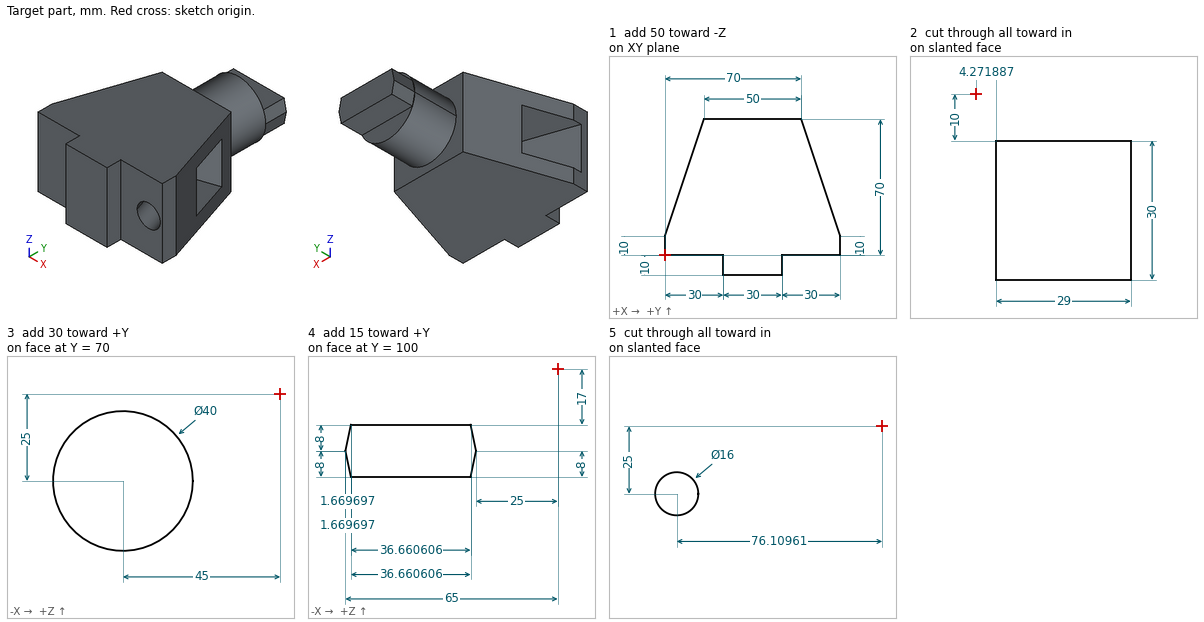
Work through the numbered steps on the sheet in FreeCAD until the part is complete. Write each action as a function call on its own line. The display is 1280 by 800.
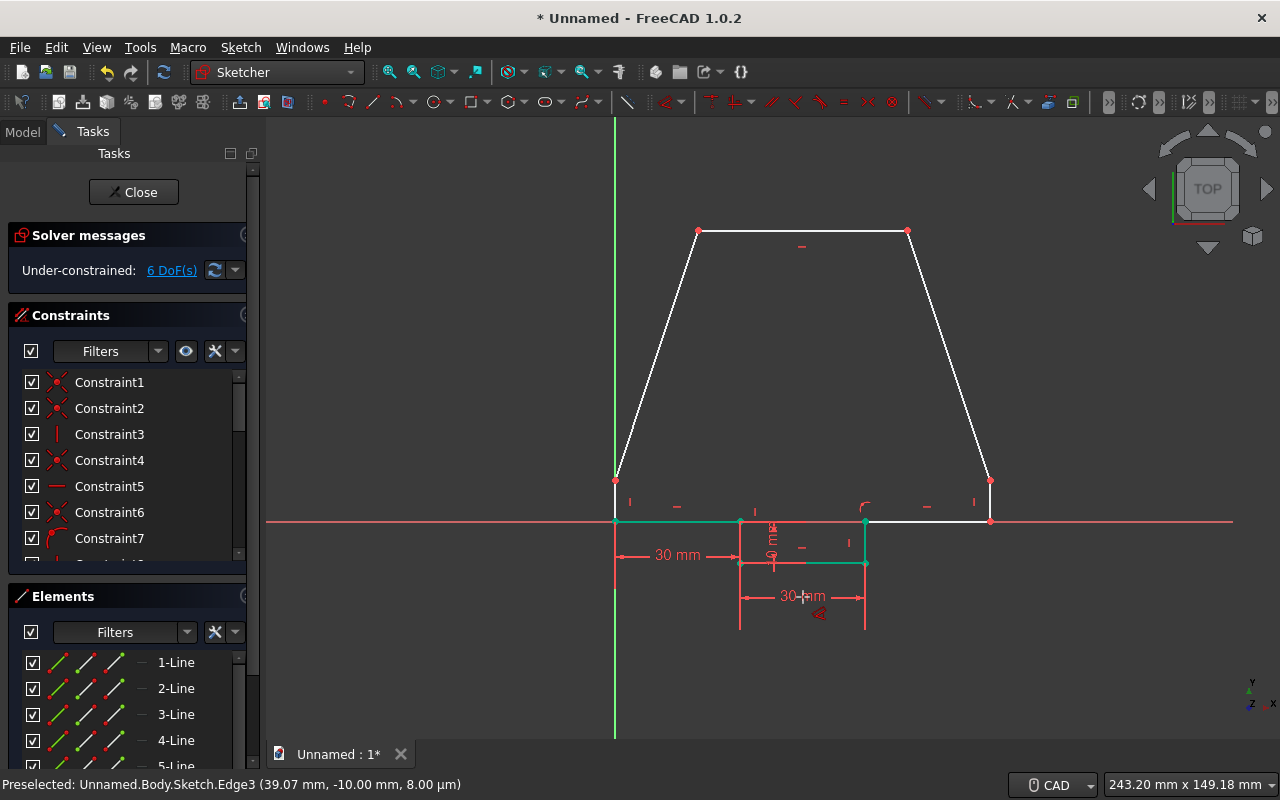
click(903, 522)
click(928, 556)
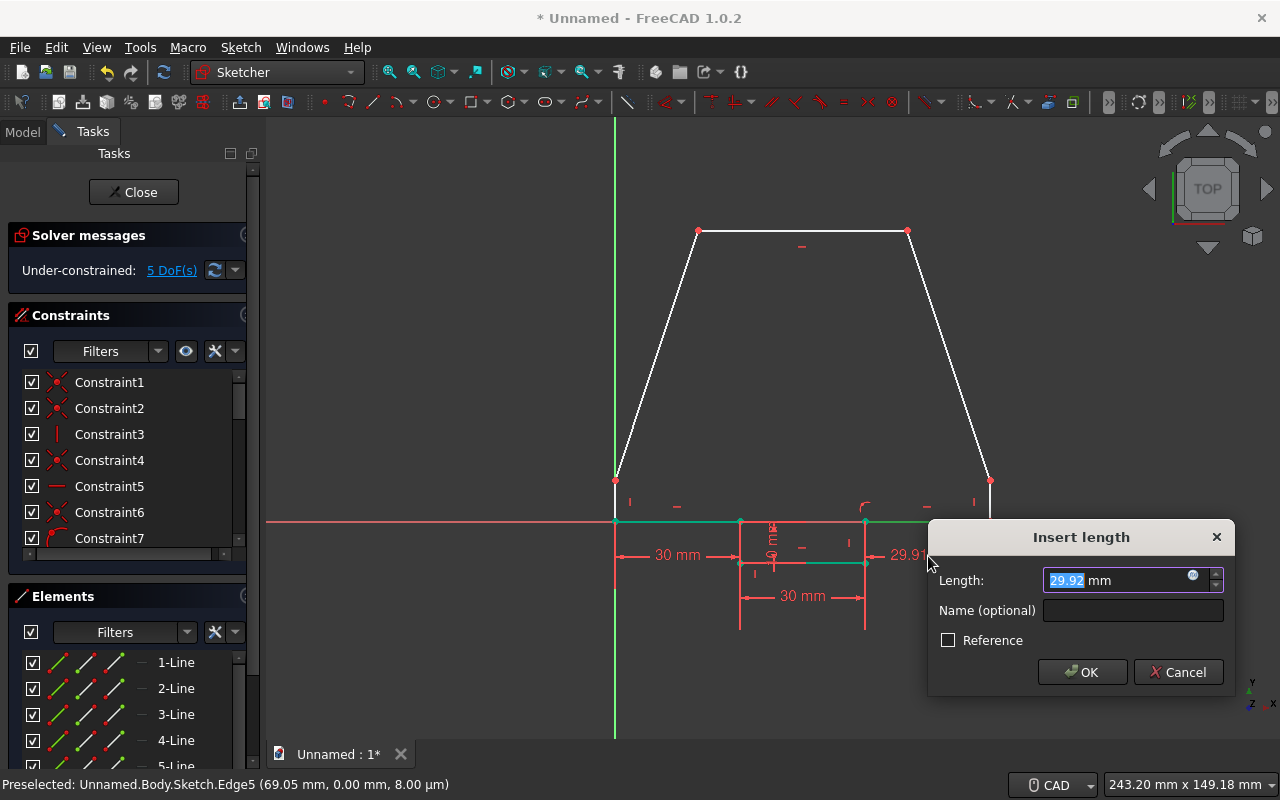
text(30)
key(Return)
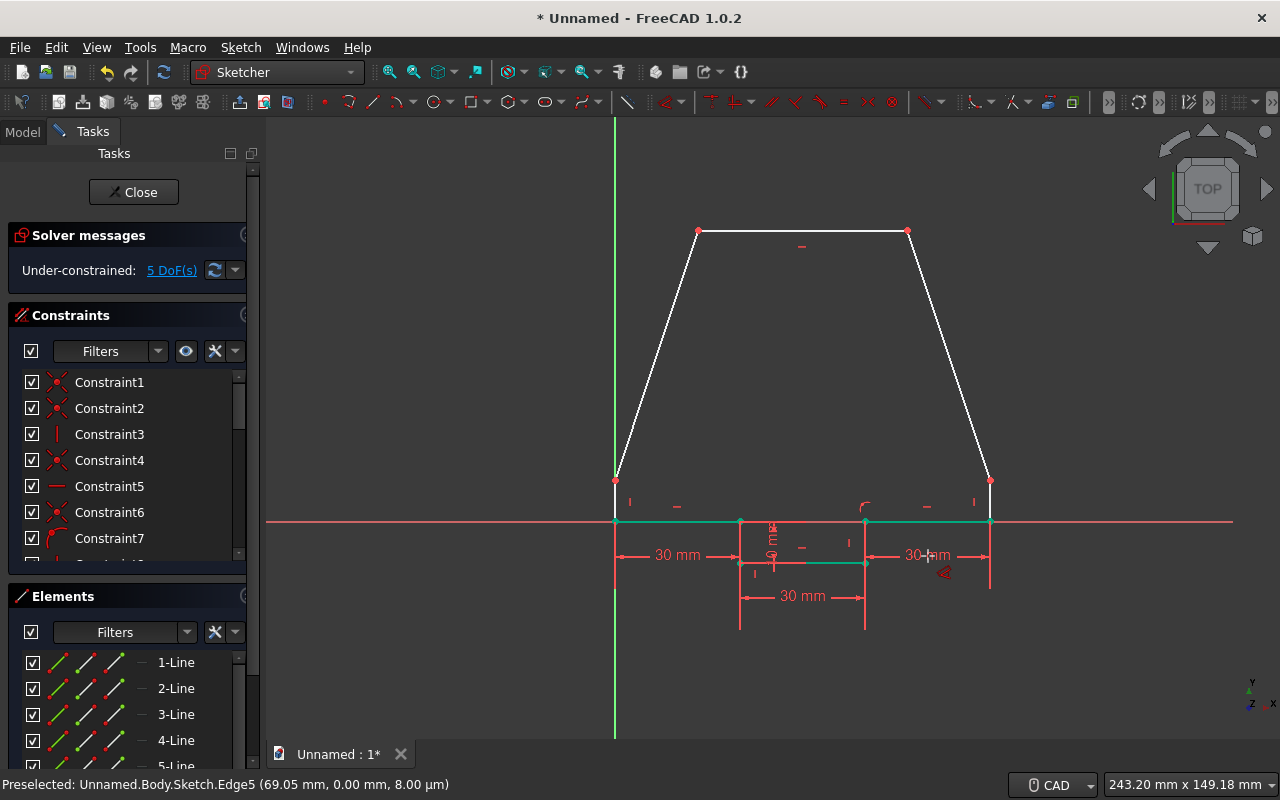
click(990, 509)
click(1024, 501)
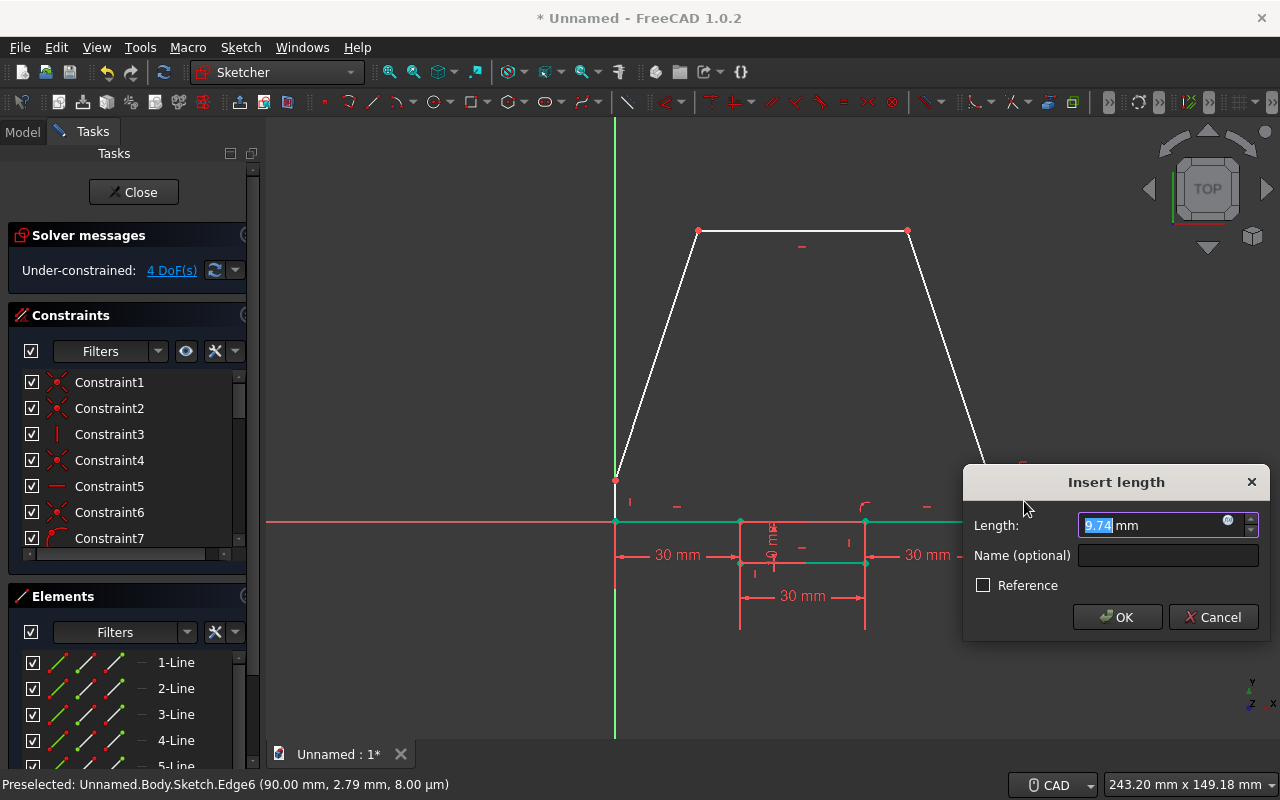
text(10)
key(Return)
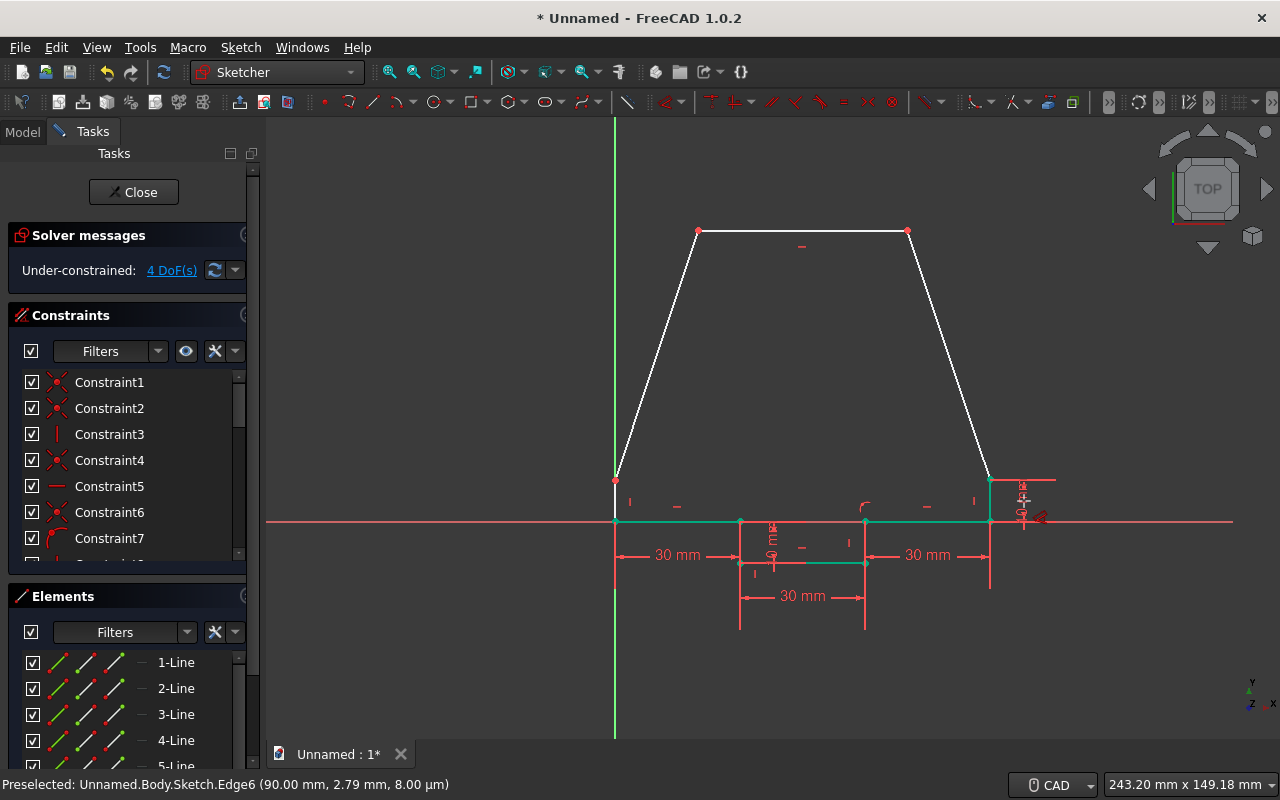
click(844, 231)
click(802, 197)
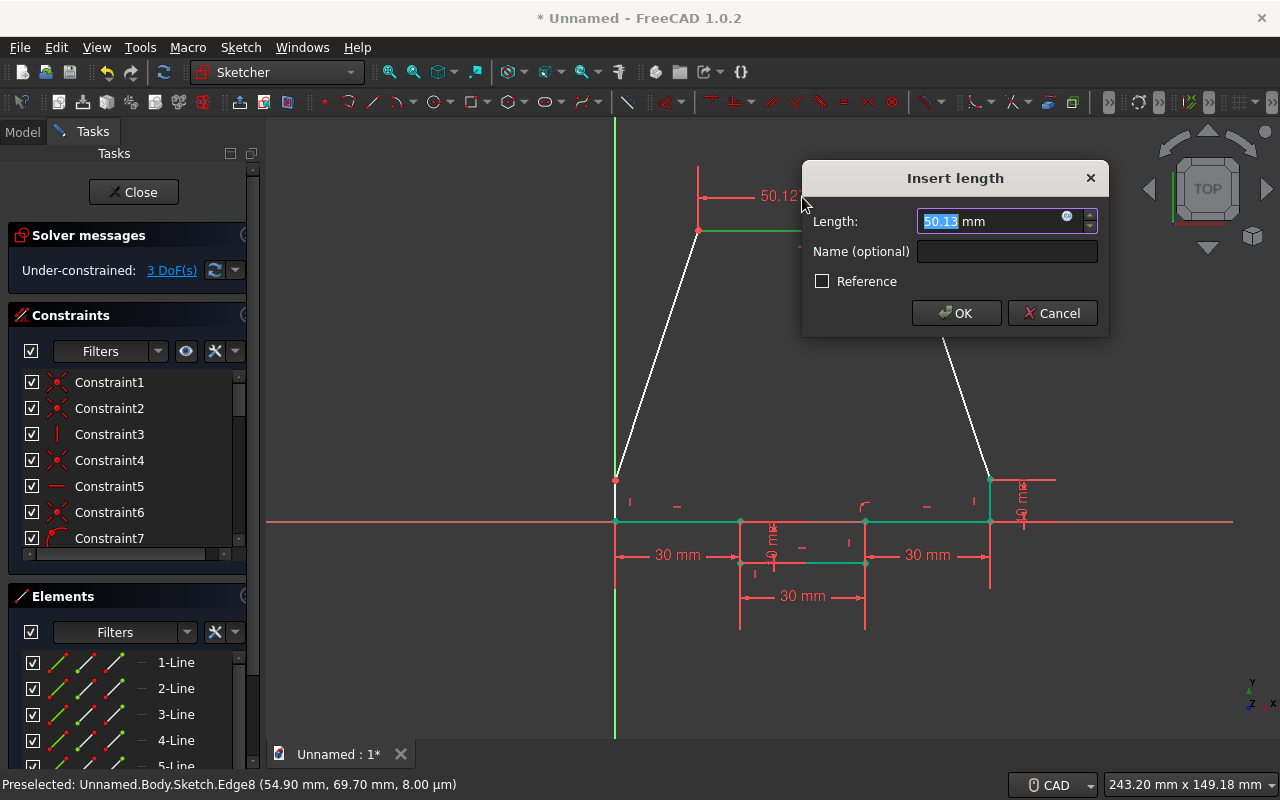
text(50)
key(Return)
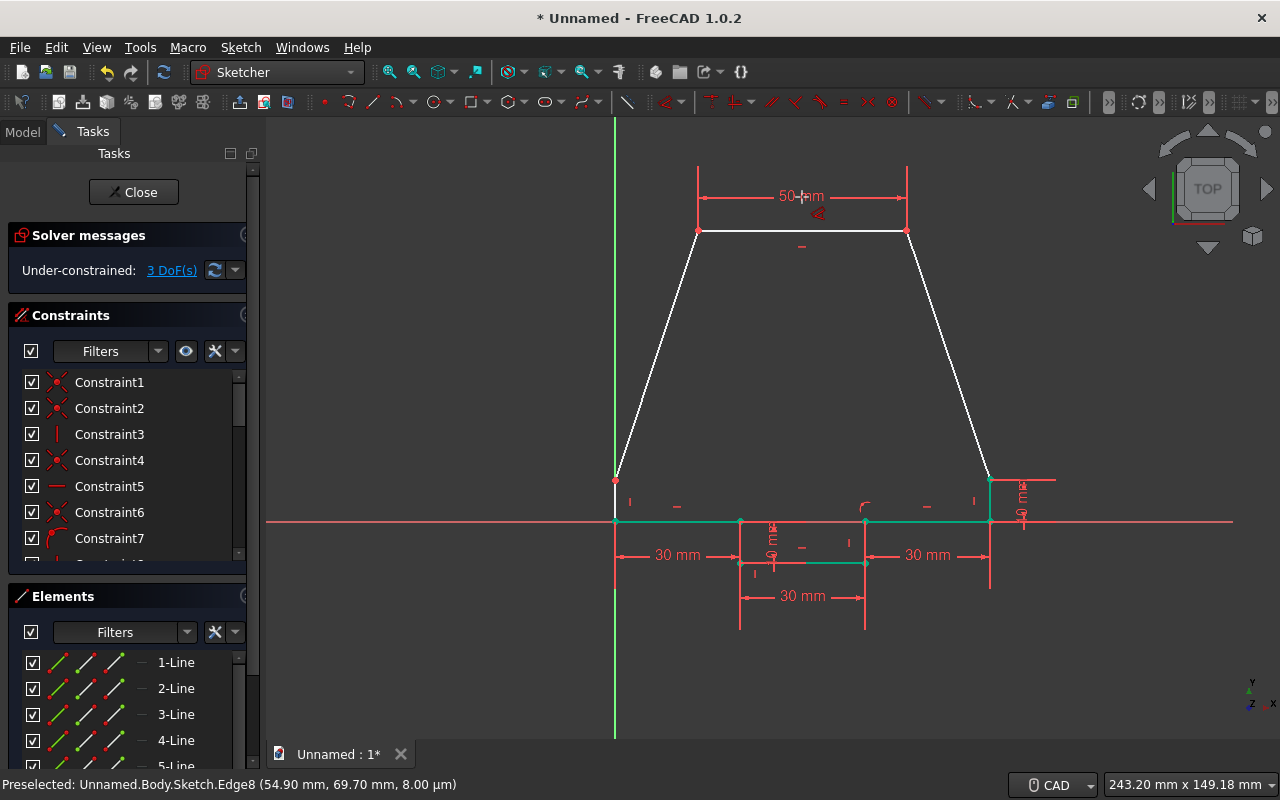
click(615, 493)
click(581, 501)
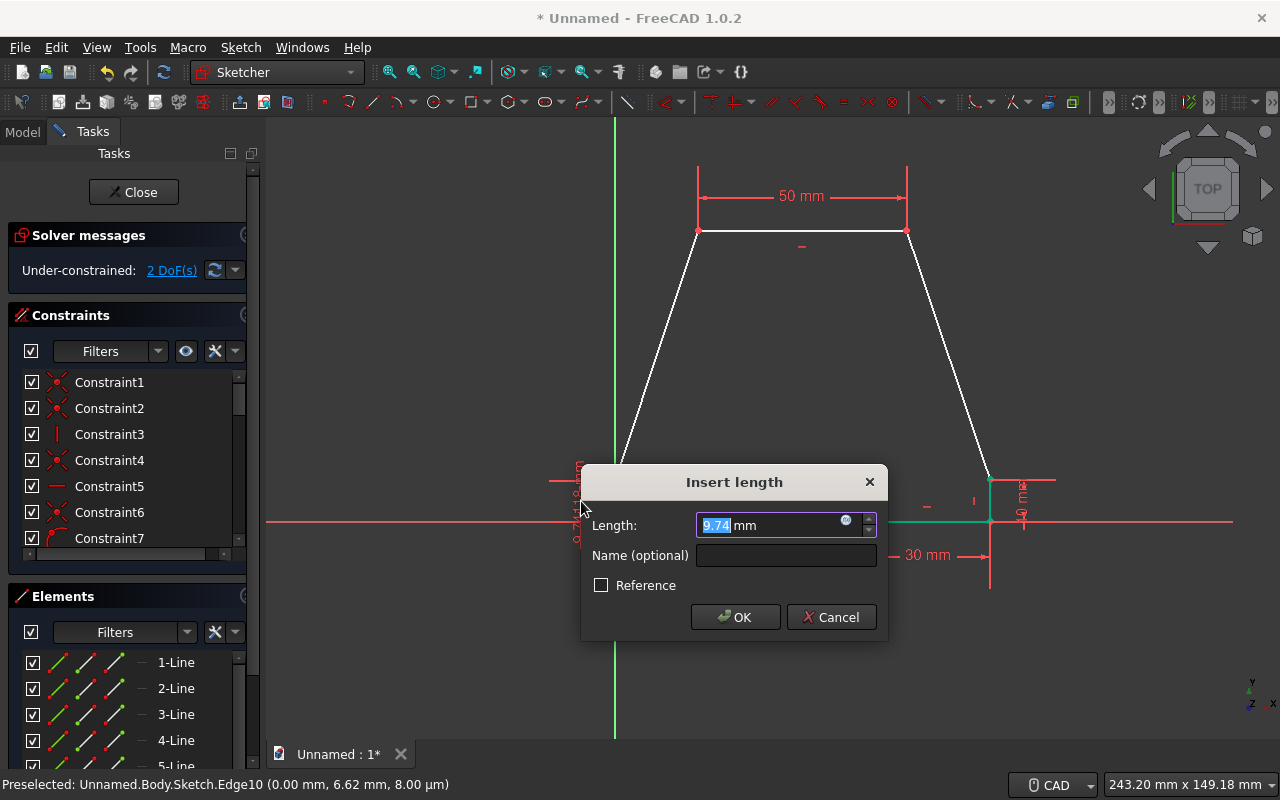
text(10)
key(Return)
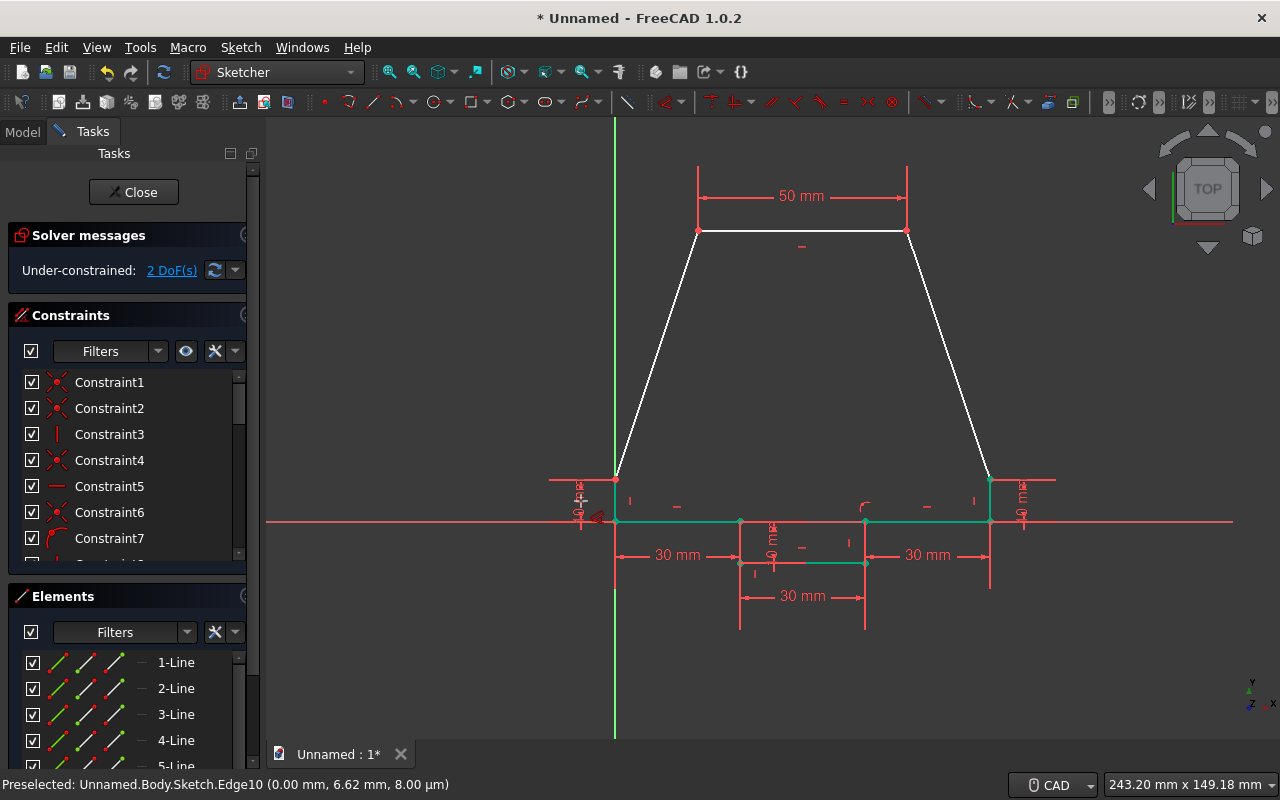
click(907, 231)
click(694, 197)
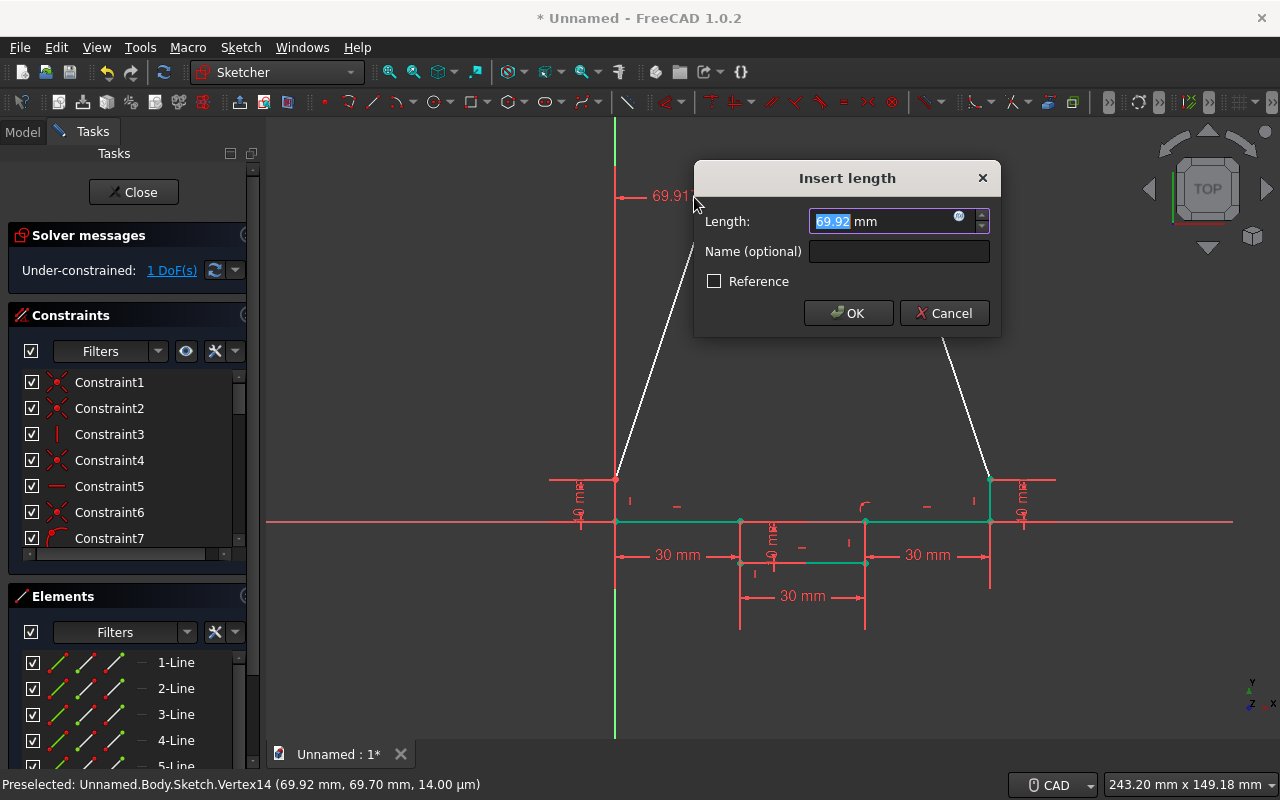
text(70)
key(Return)